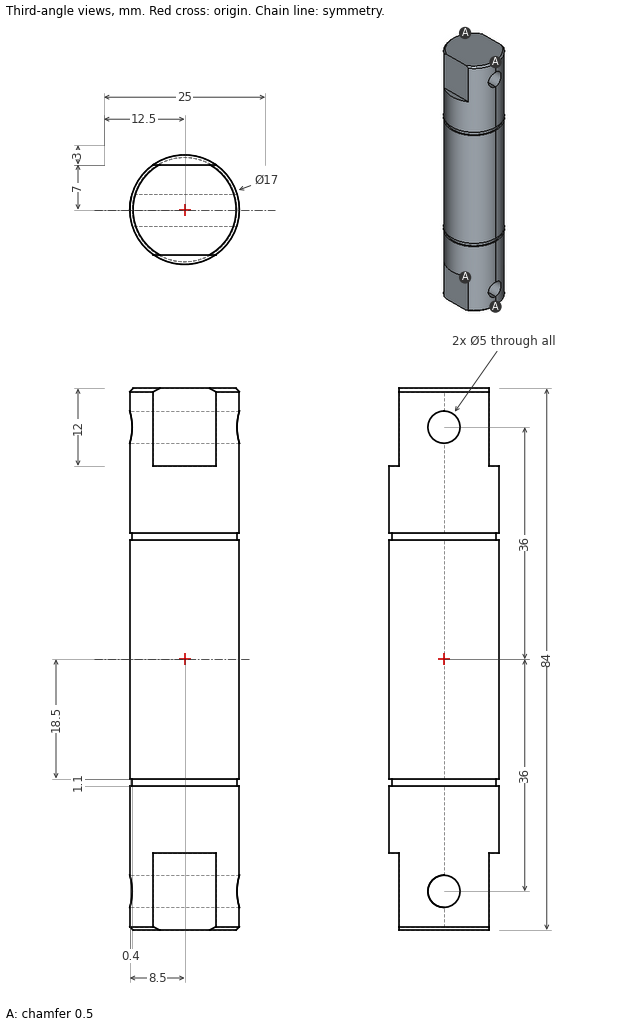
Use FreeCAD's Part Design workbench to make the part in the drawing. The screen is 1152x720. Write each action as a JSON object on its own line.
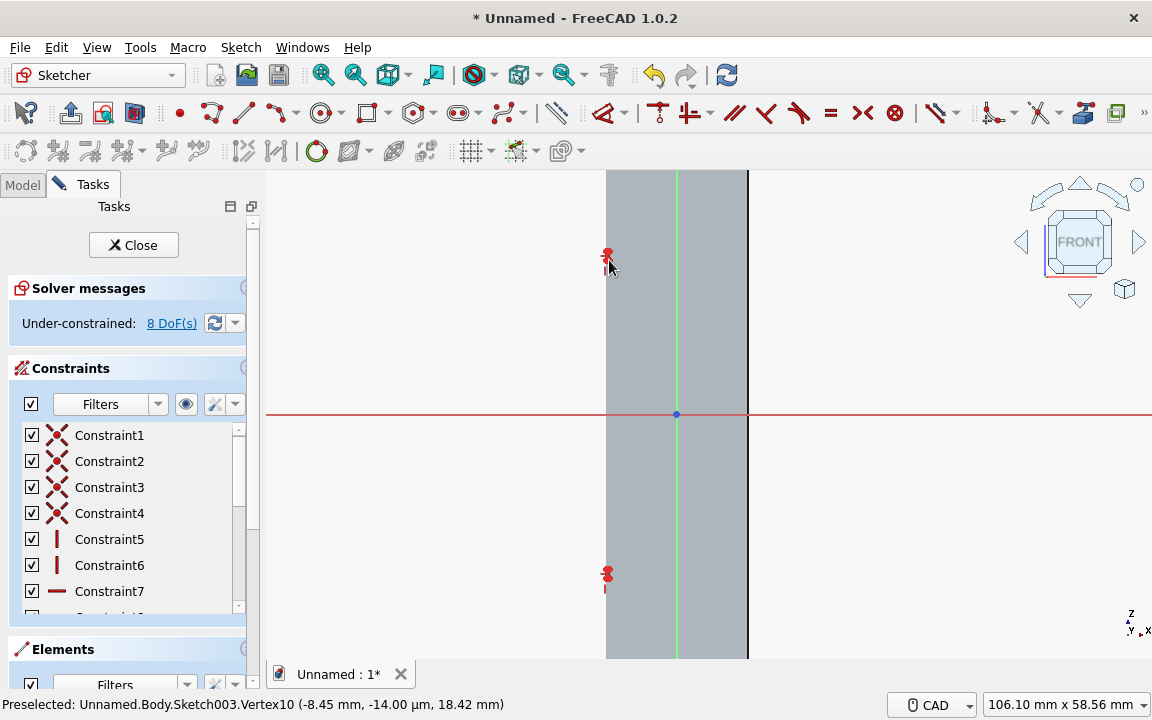
{"action": "scroll", "coordinate": [606, 579], "scroll_direction": "up", "scroll_amount": 8}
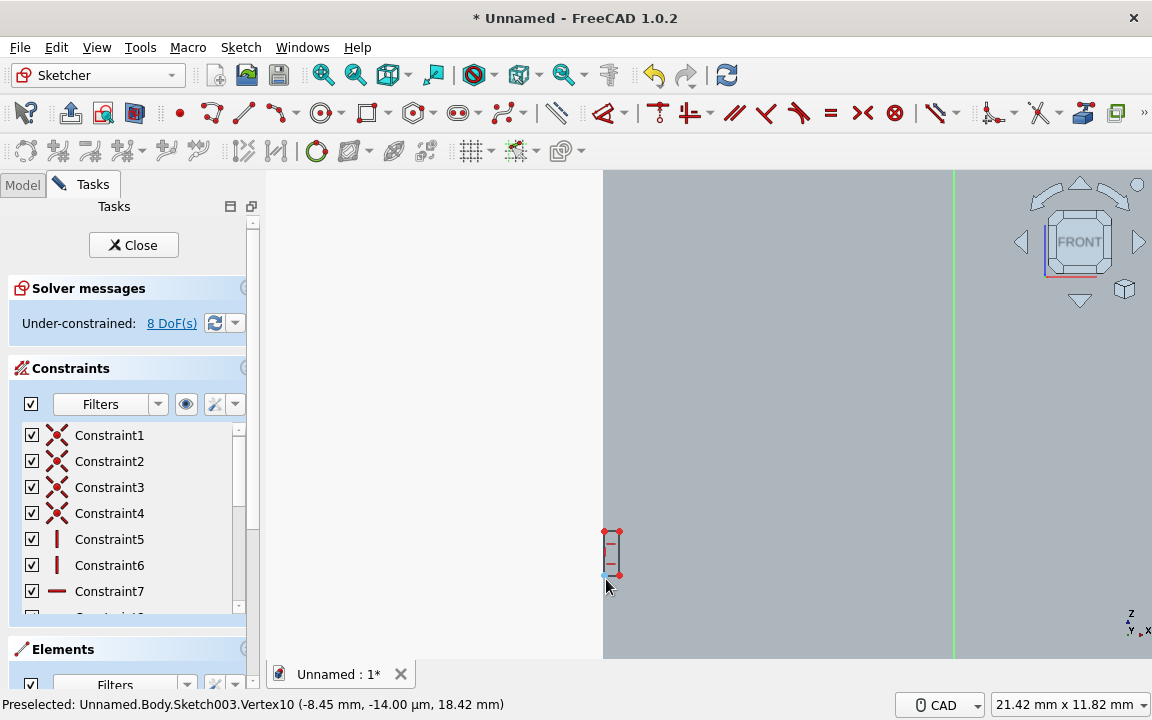
{"action": "left_click", "coordinate": [604, 576]}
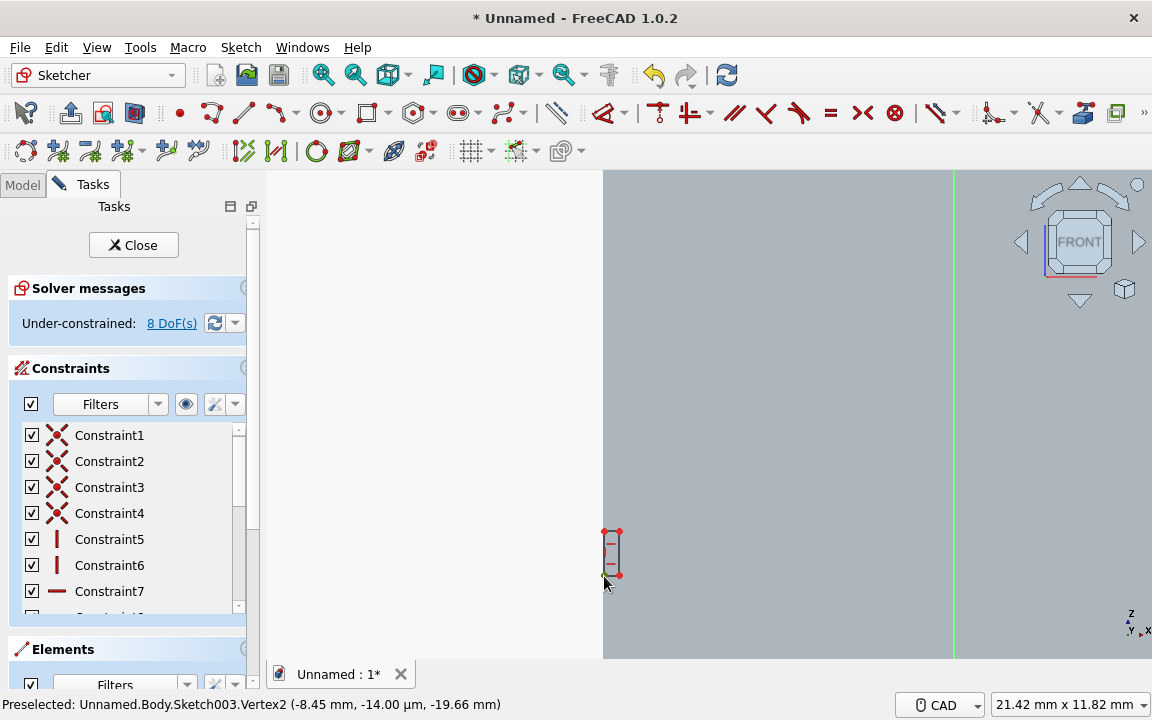
{"action": "scroll", "coordinate": [606, 579], "scroll_direction": "down", "scroll_amount": 8}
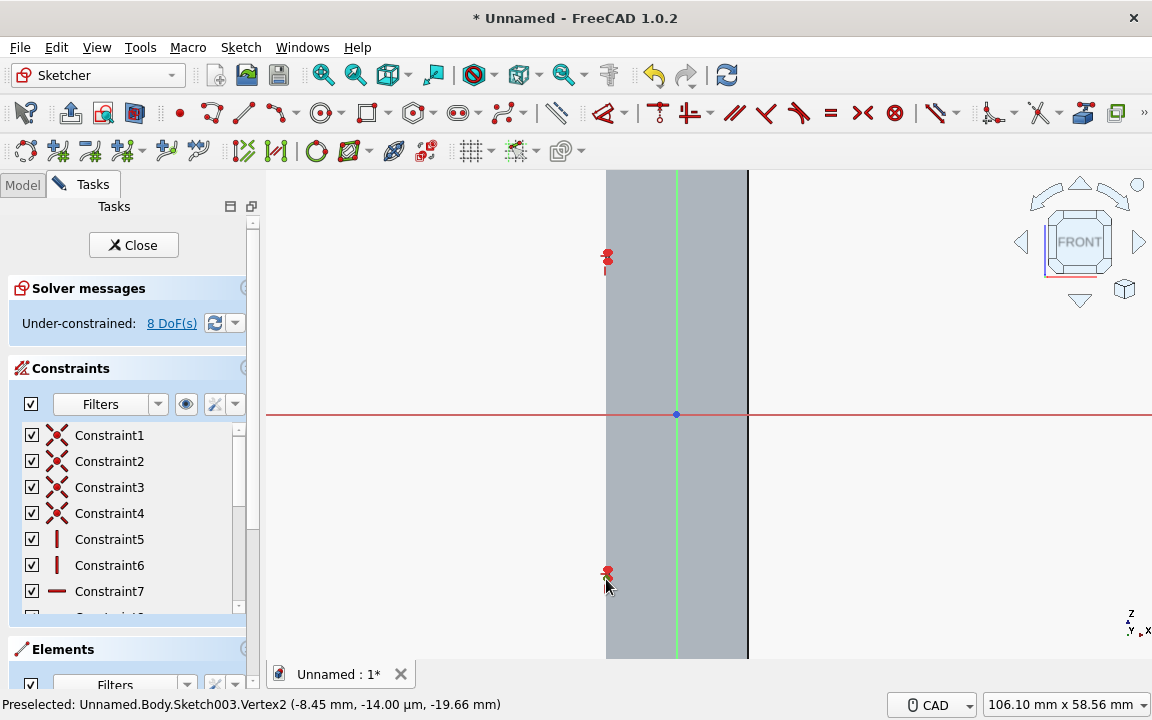
{"action": "scroll", "coordinate": [606, 252], "scroll_direction": "up", "scroll_amount": 8}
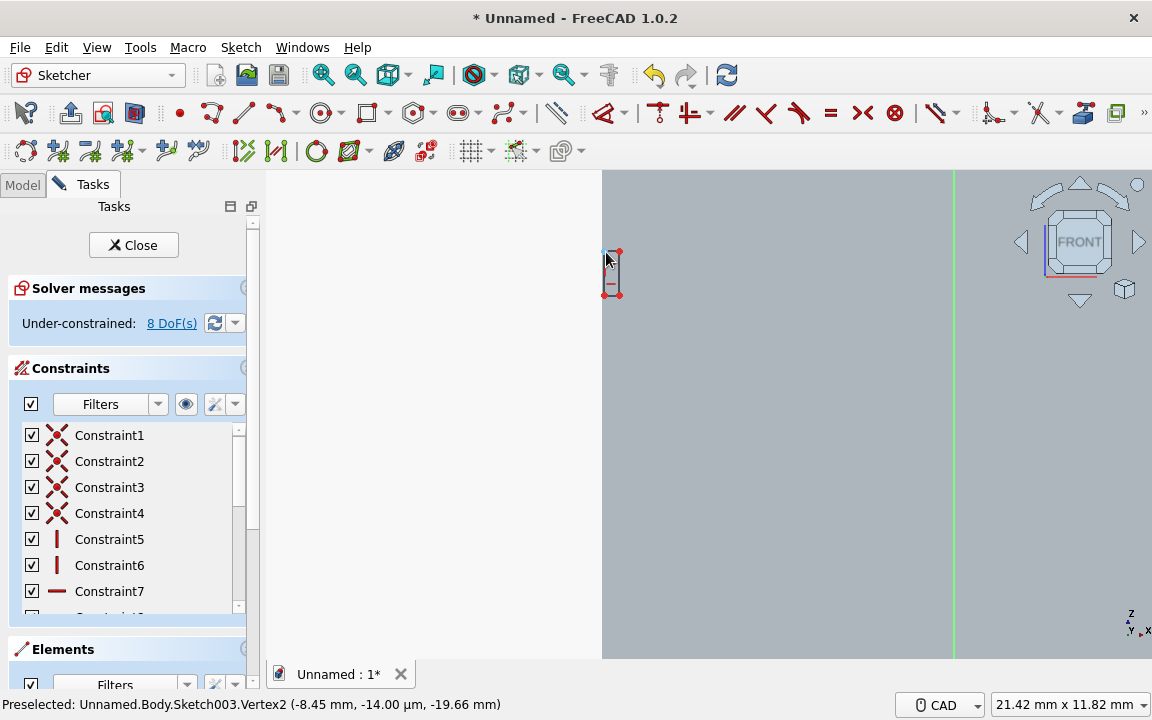
{"action": "left_click", "coordinate": [604, 251]}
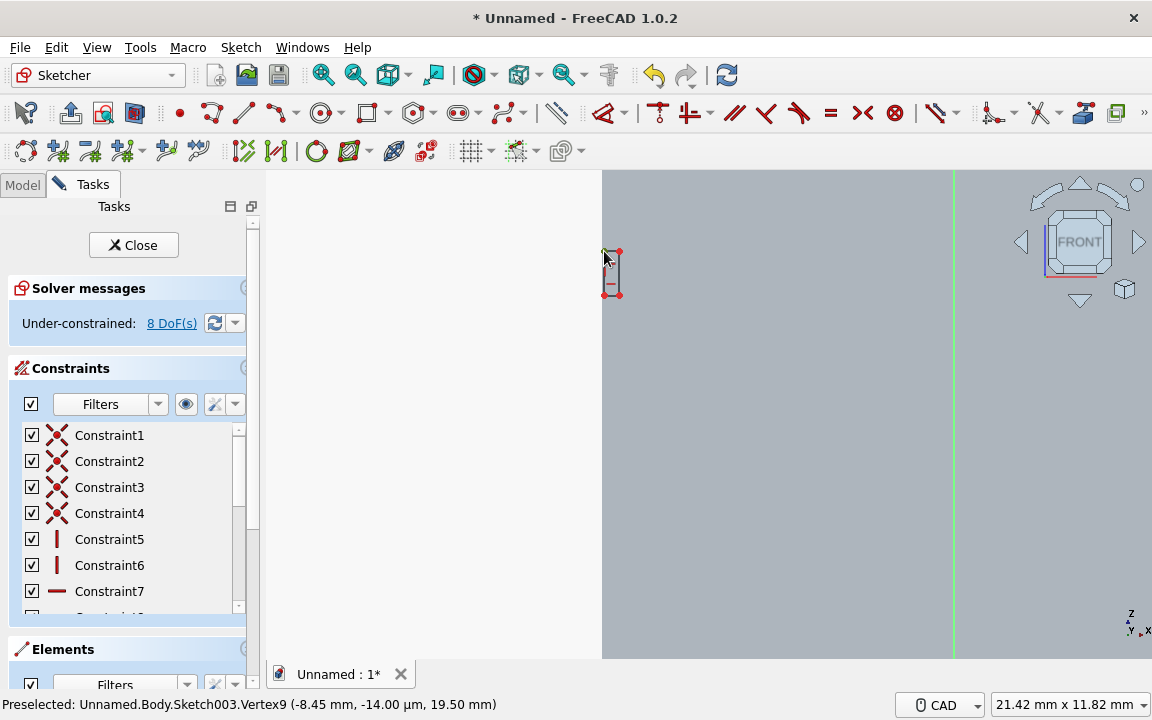
{"action": "scroll", "coordinate": [606, 252], "scroll_direction": "down", "scroll_amount": 8}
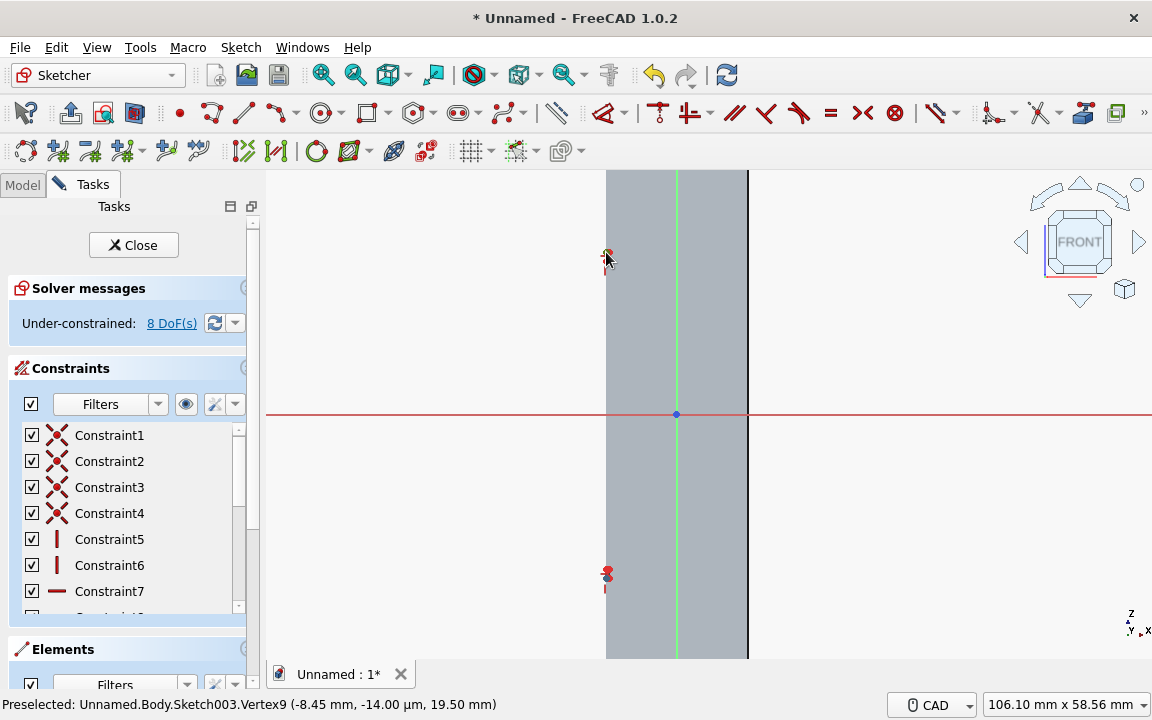
{"action": "left_click", "coordinate": [344, 415]}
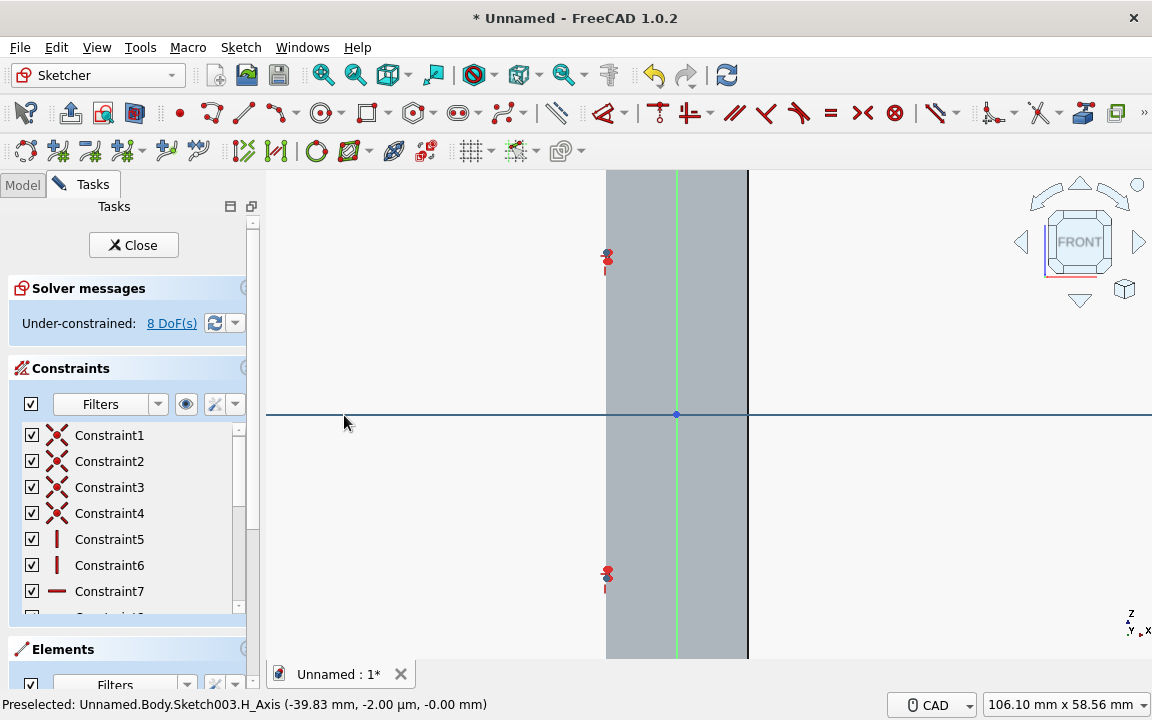
{"action": "left_click", "coordinate": [864, 114]}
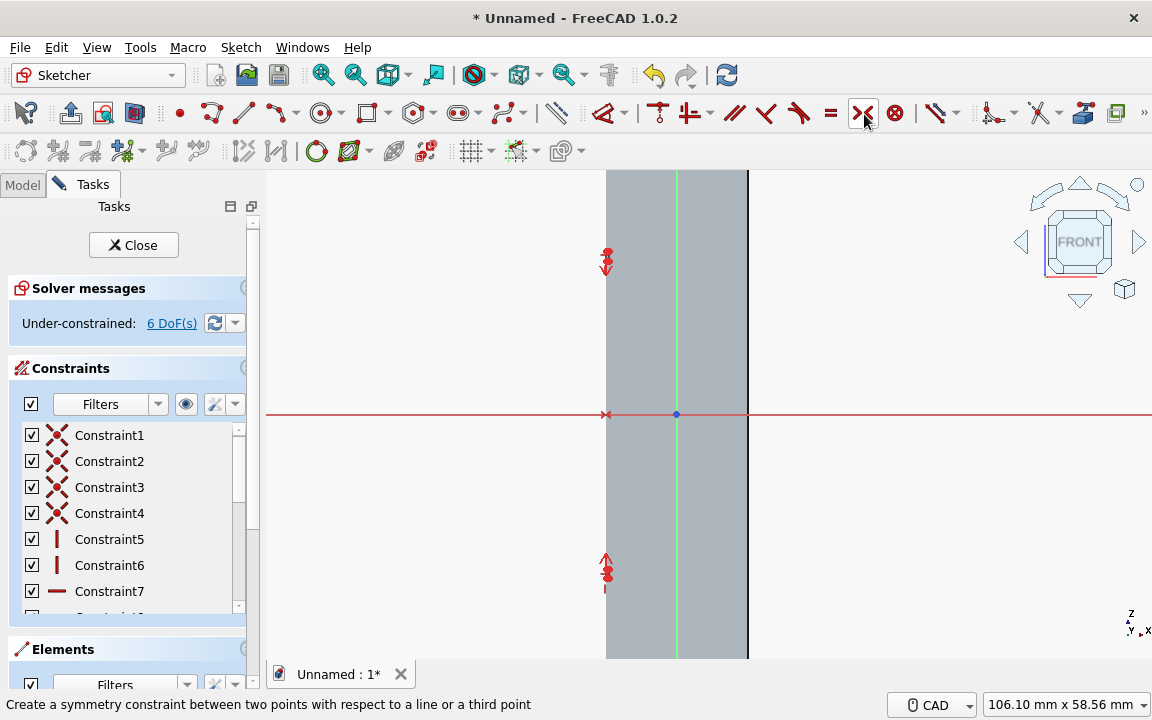
{"action": "scroll", "coordinate": [609, 570], "scroll_direction": "up", "scroll_amount": 8}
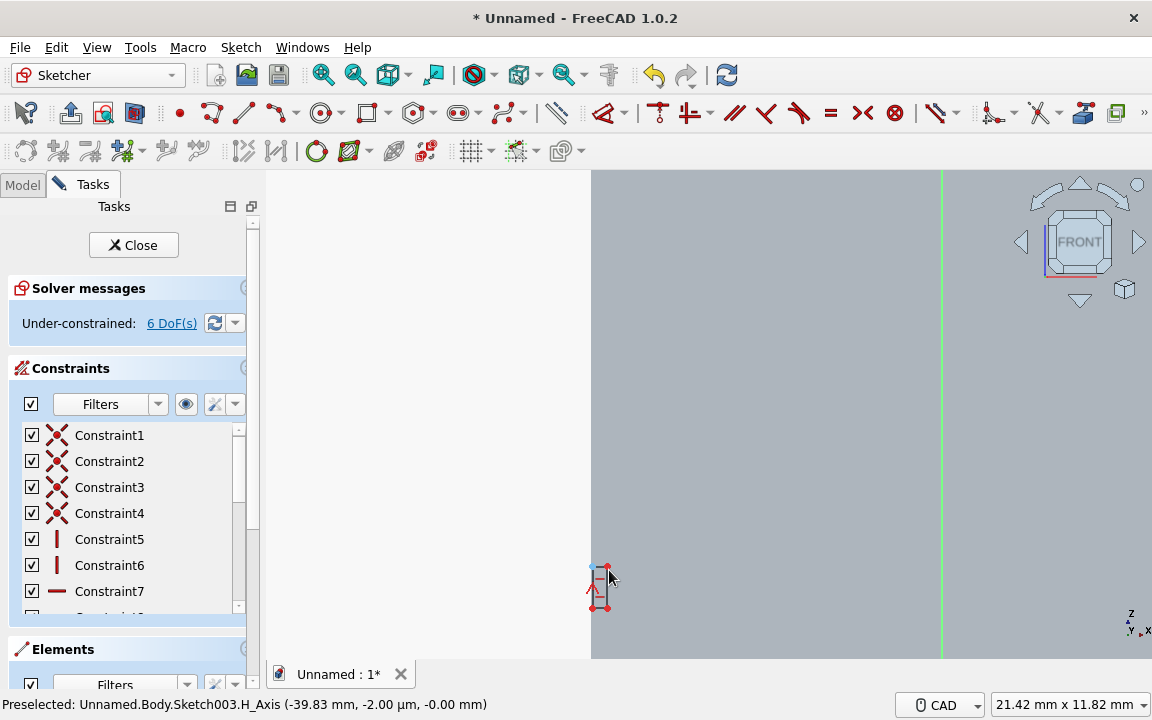
{"action": "left_click", "coordinate": [607, 567]}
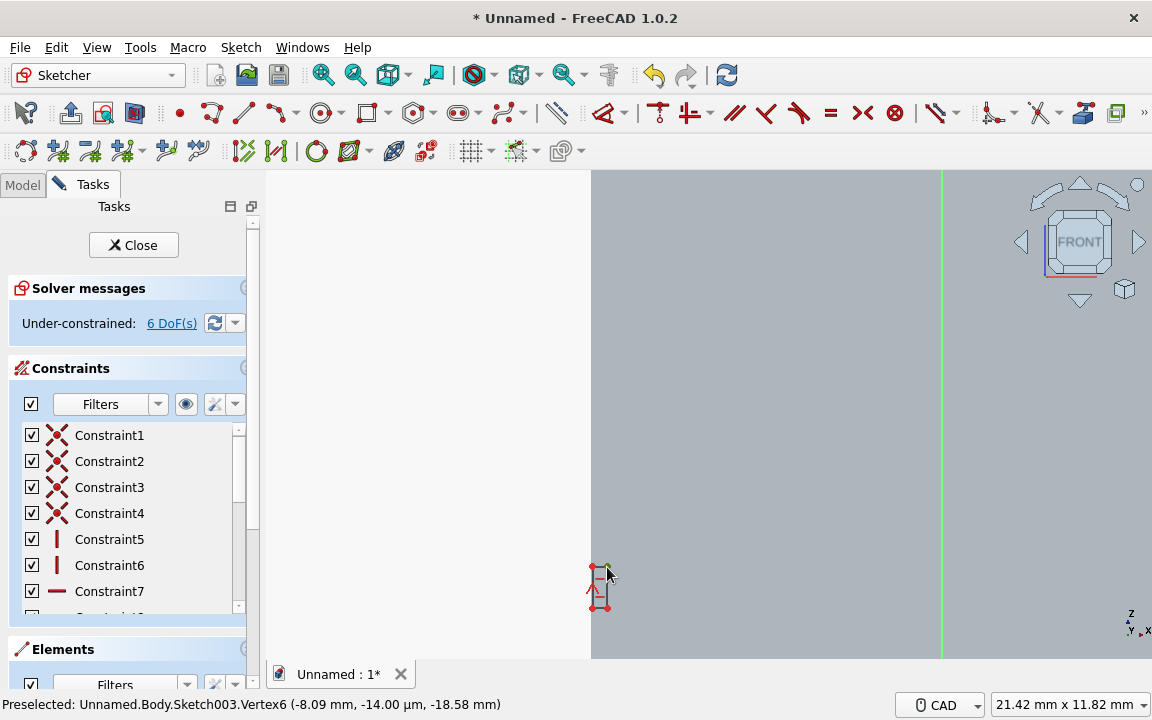
{"action": "scroll", "coordinate": [609, 570], "scroll_direction": "down", "scroll_amount": 8}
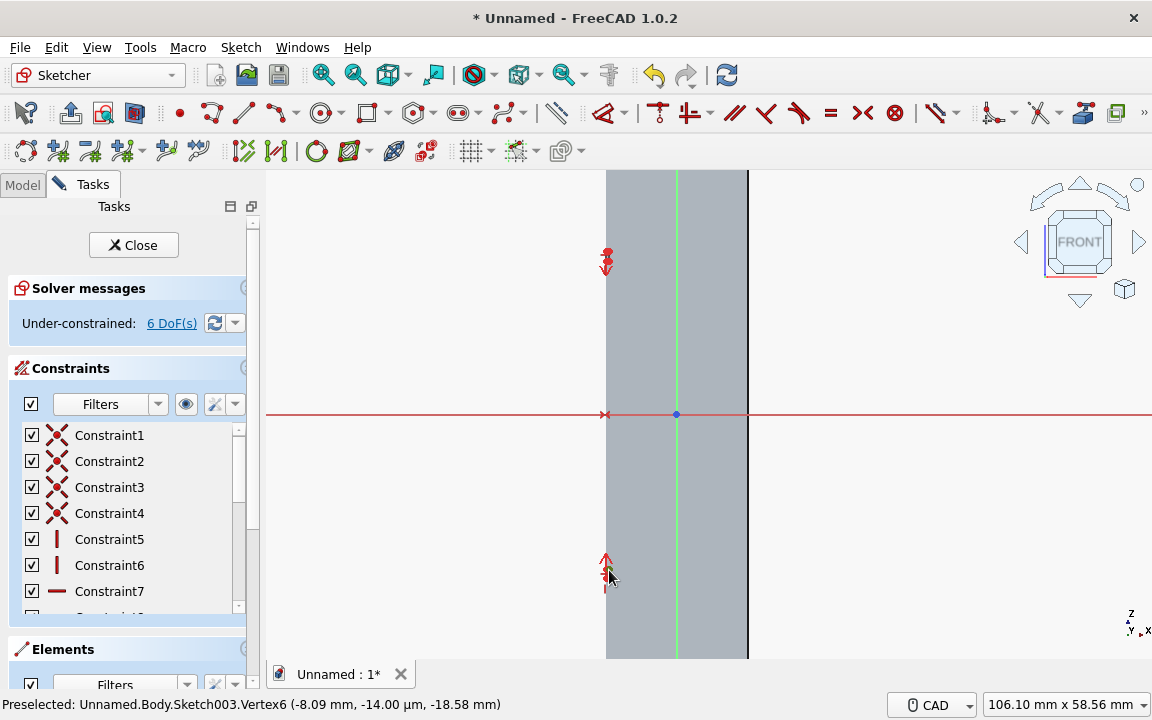
{"action": "scroll", "coordinate": [609, 261], "scroll_direction": "up", "scroll_amount": 8}